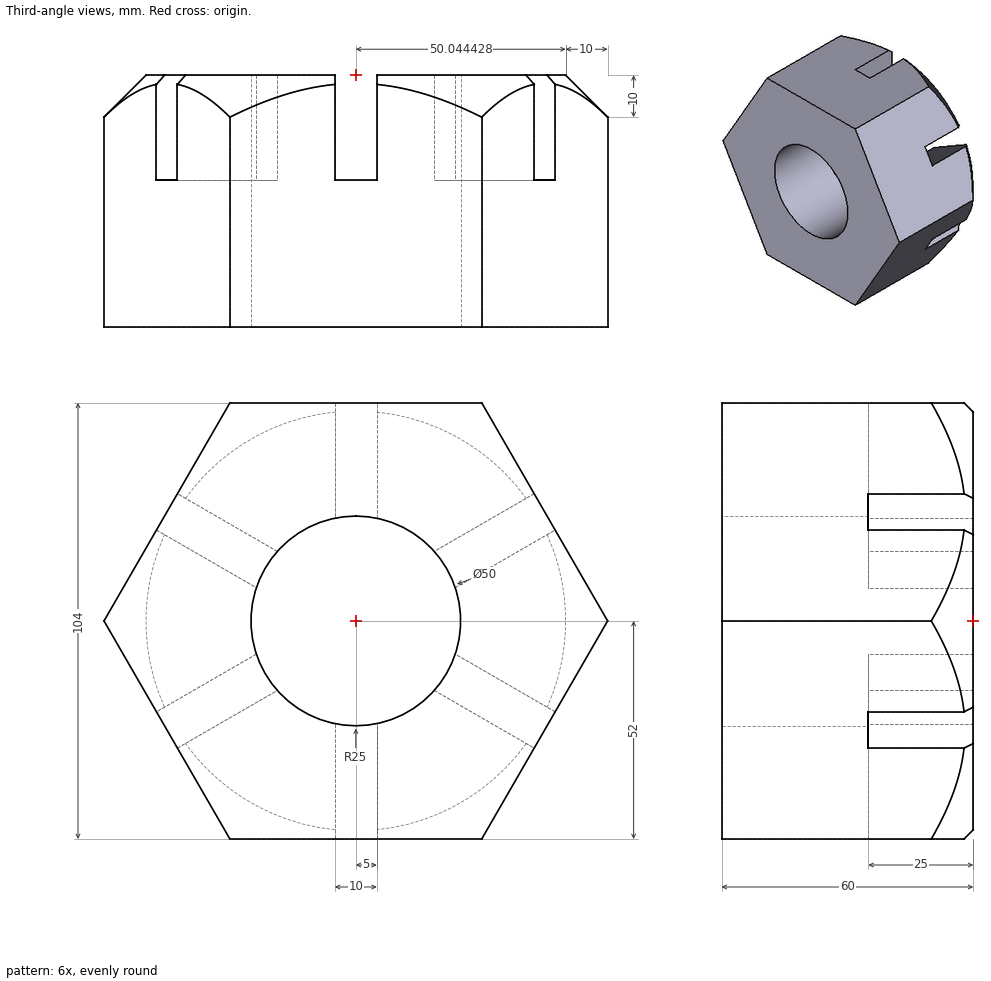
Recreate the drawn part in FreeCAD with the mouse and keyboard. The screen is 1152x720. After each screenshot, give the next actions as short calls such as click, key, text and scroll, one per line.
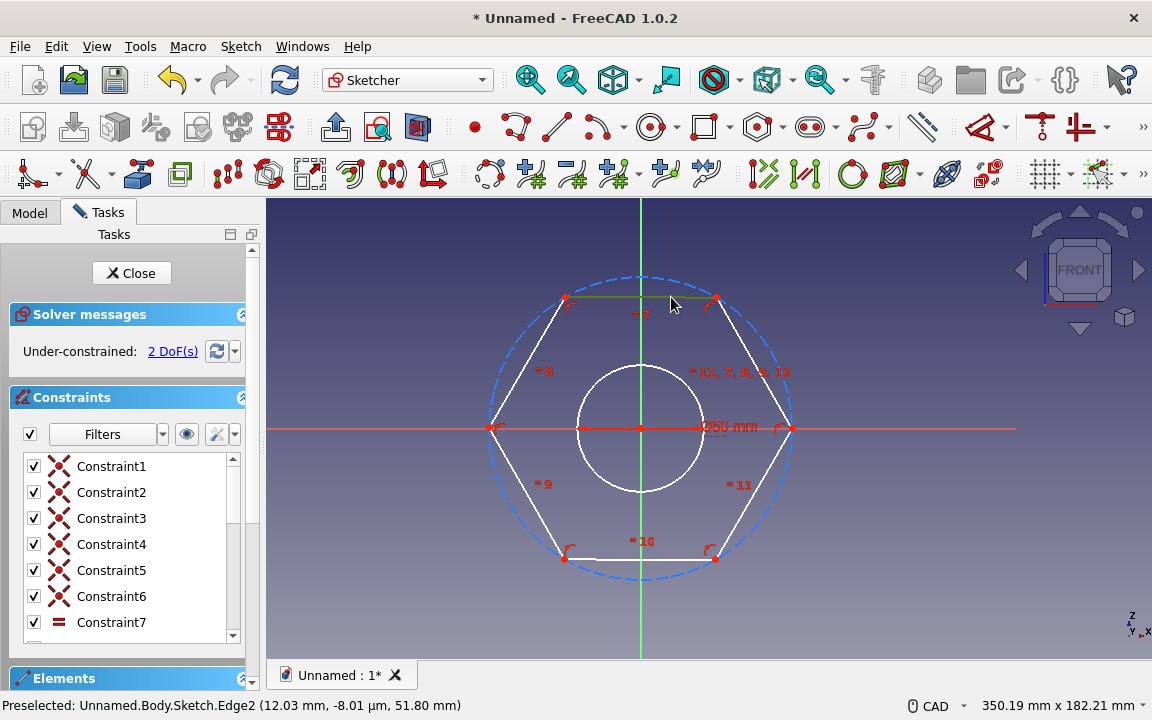
key(h)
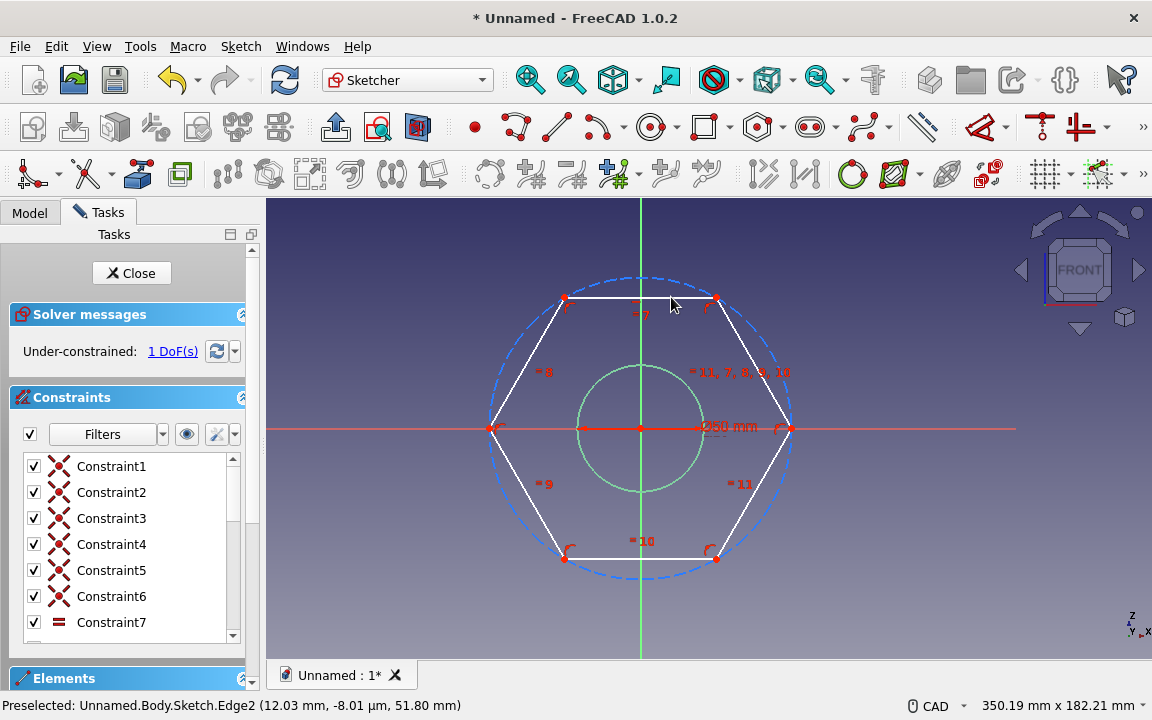
click(980, 128)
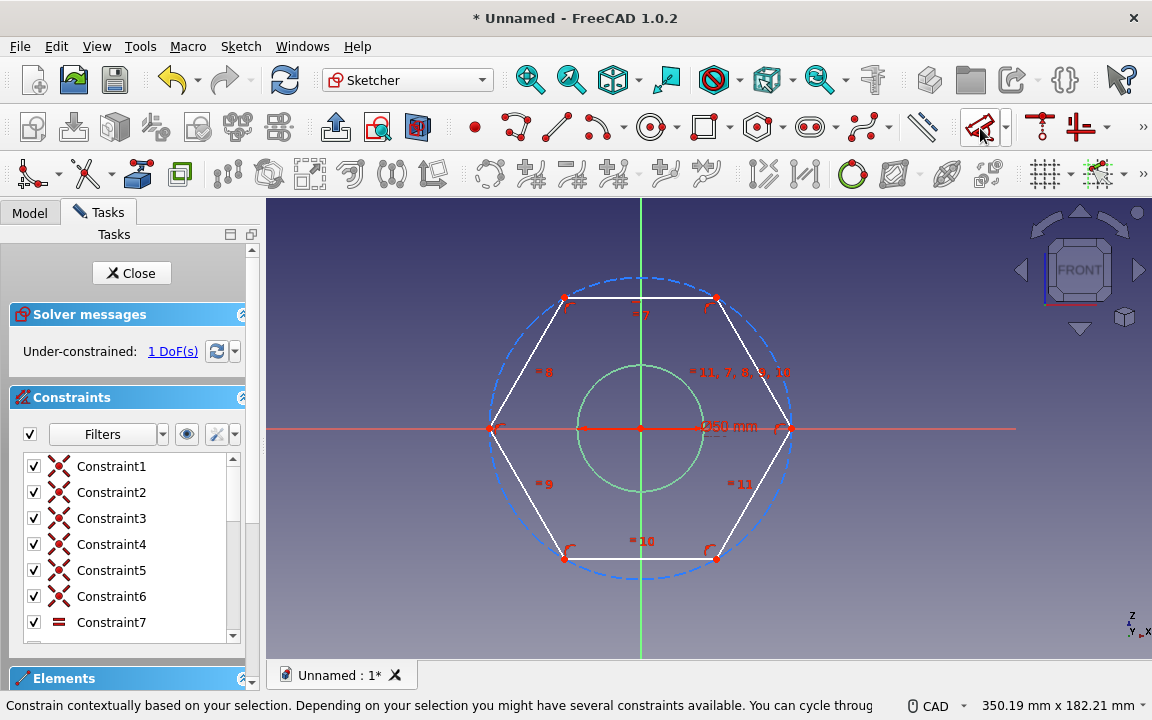
click(565, 559)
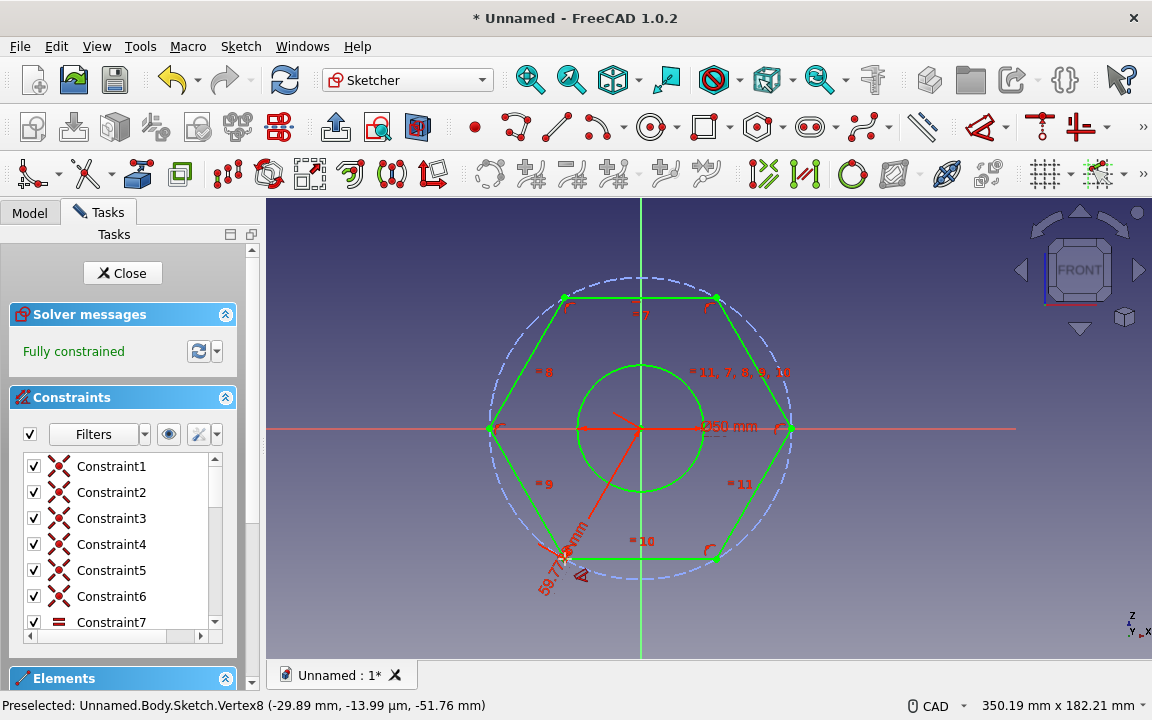
click(716, 298)
click(483, 368)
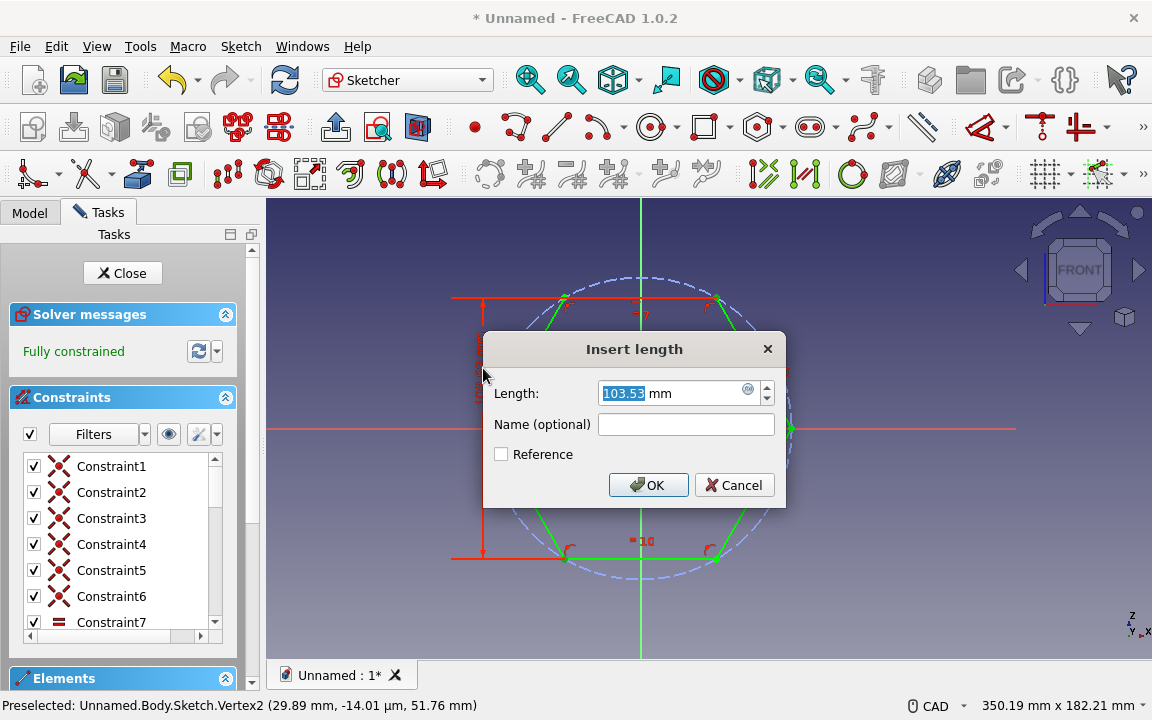
text(104)
key(Return)
key(Escape)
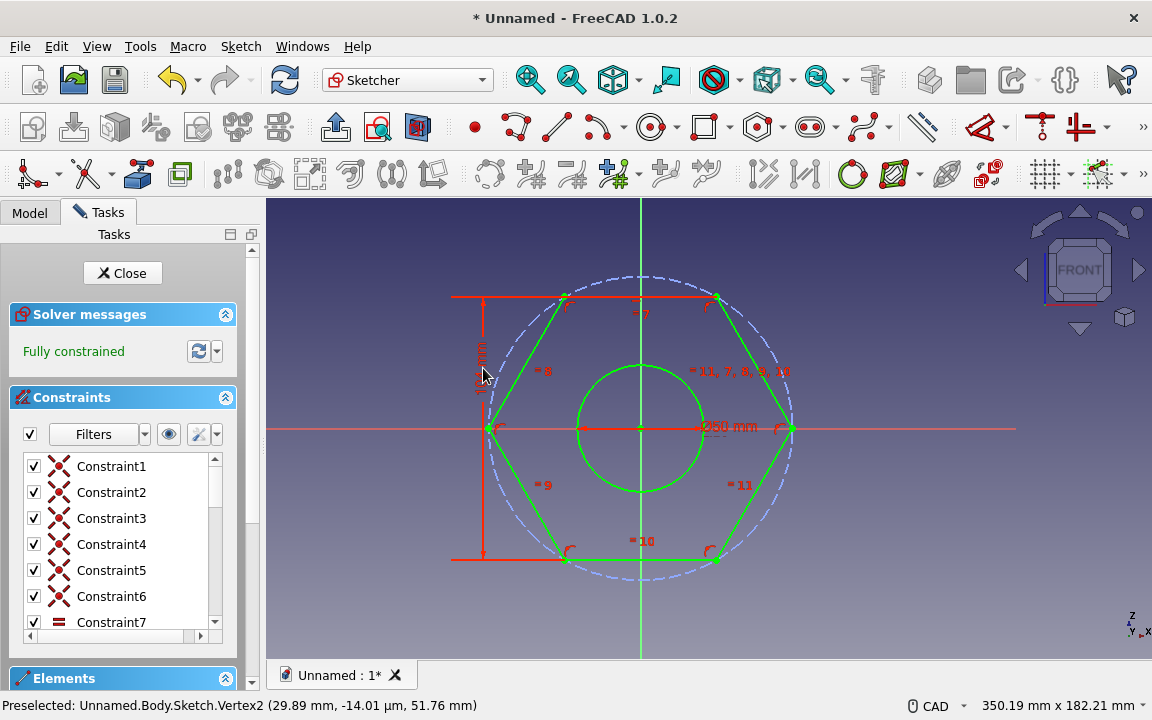
click(123, 273)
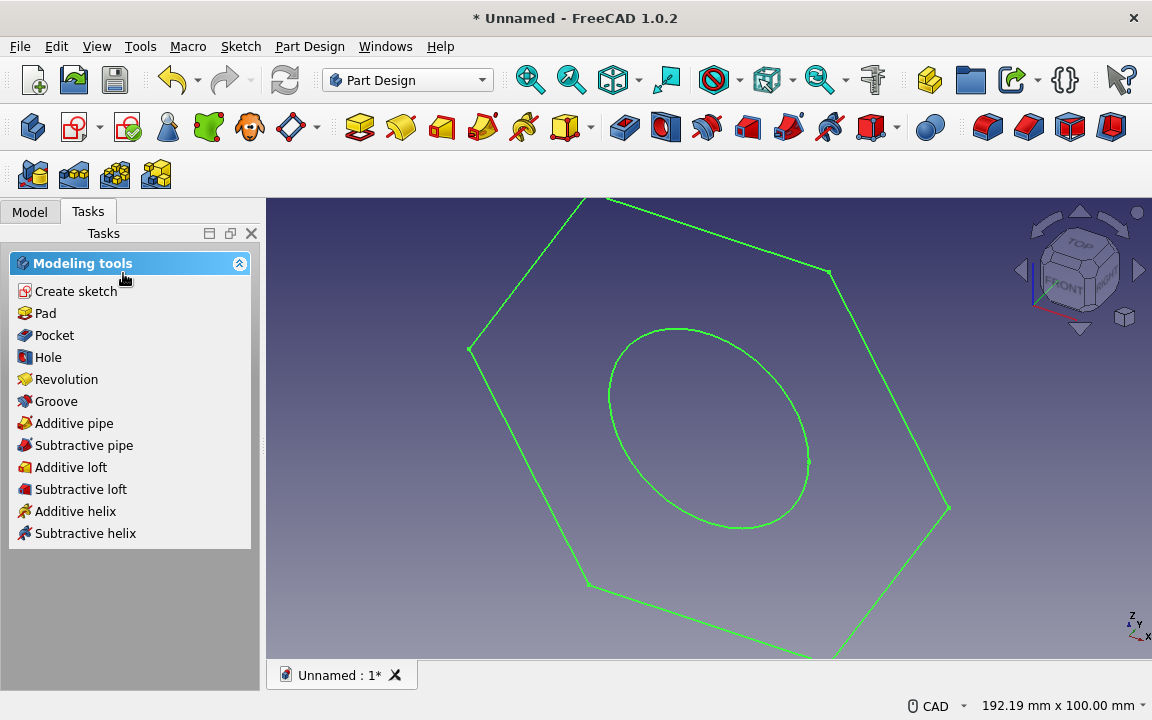
click(360, 128)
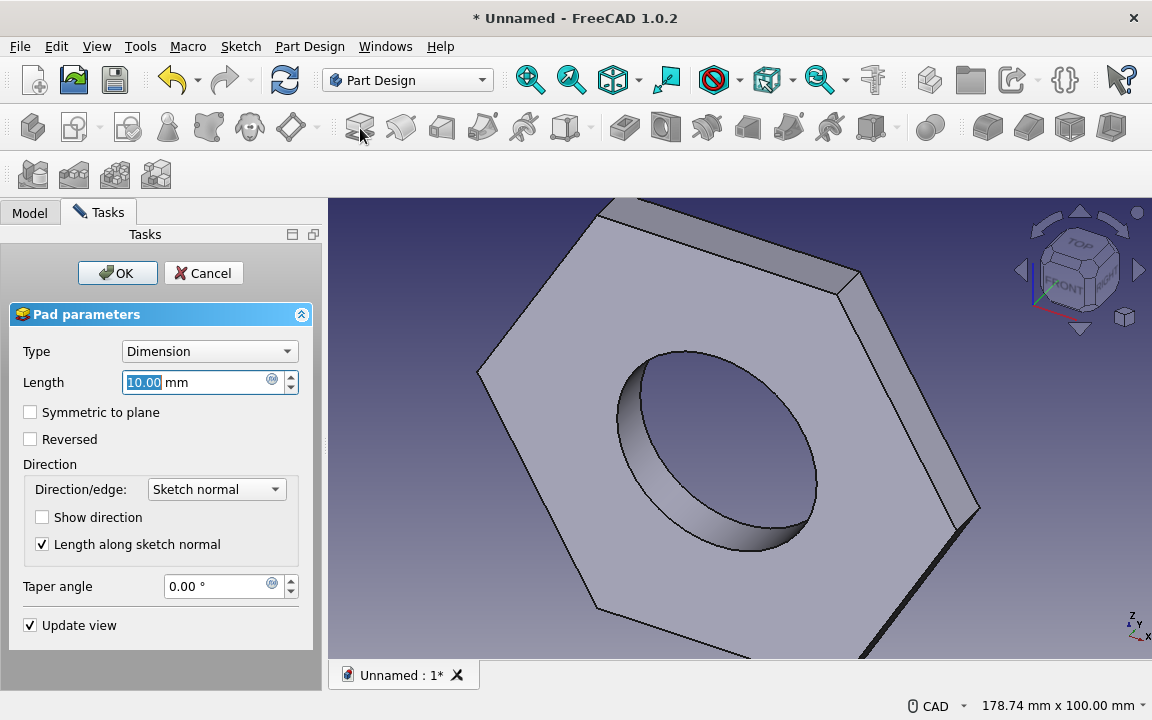
text(60)
key(Tab)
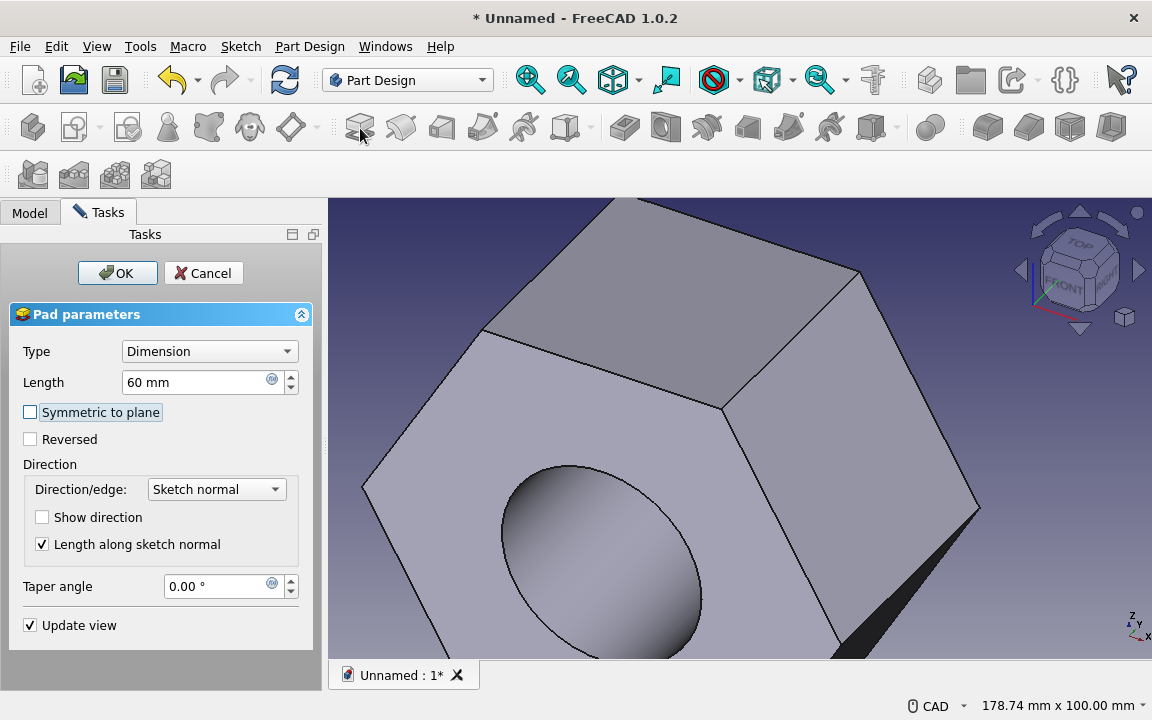
click(118, 273)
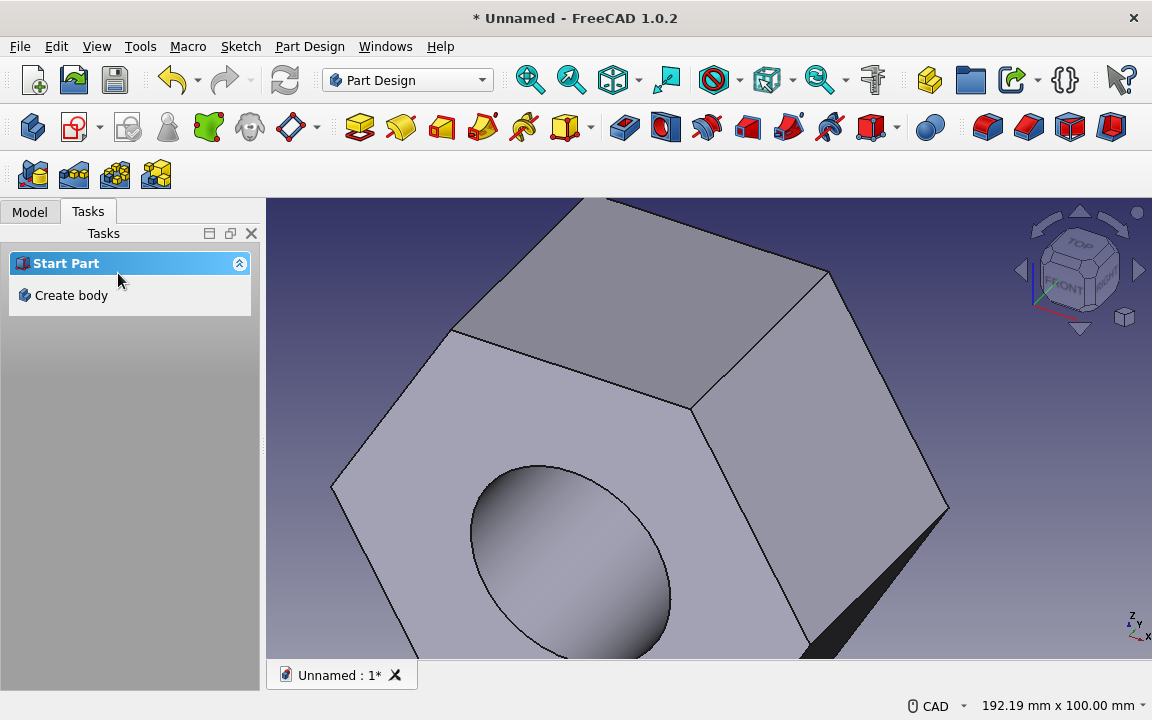
click(531, 80)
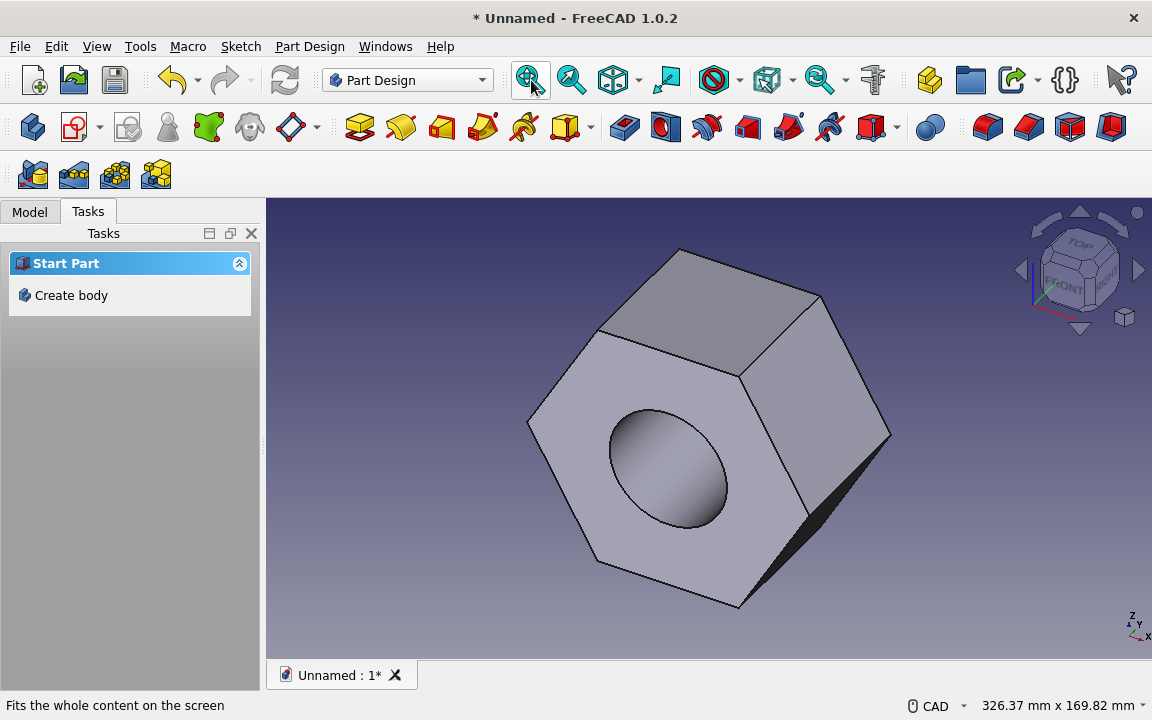
click(74, 128)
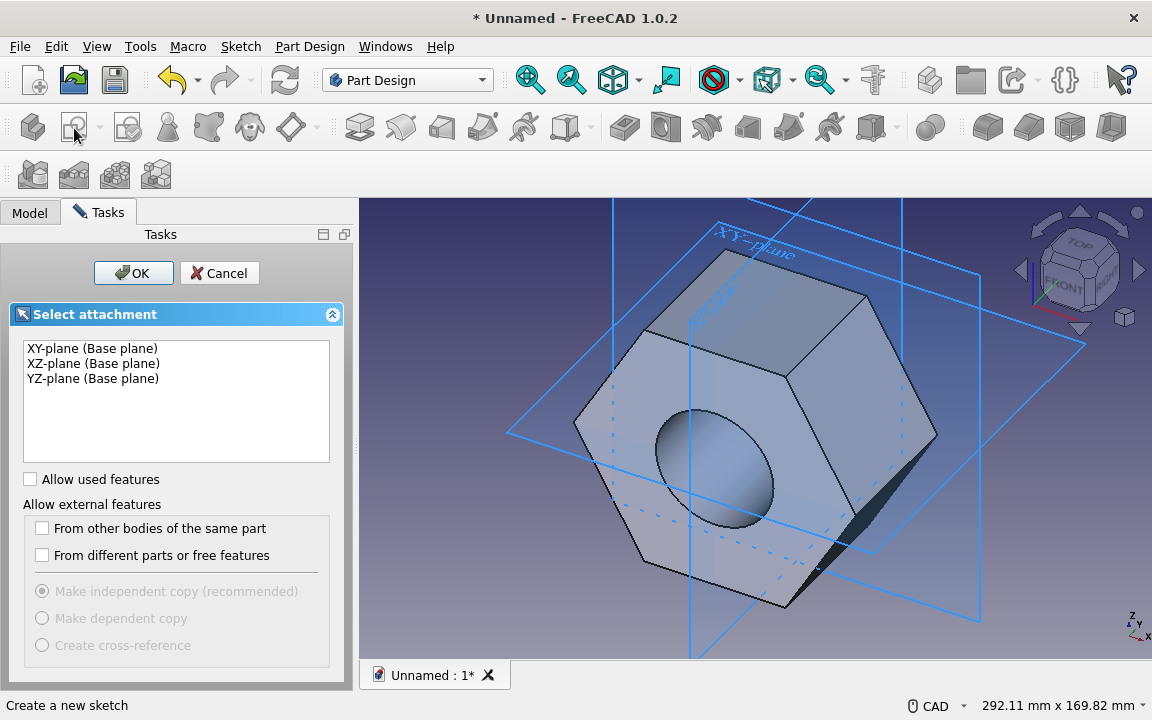
click(84, 348)